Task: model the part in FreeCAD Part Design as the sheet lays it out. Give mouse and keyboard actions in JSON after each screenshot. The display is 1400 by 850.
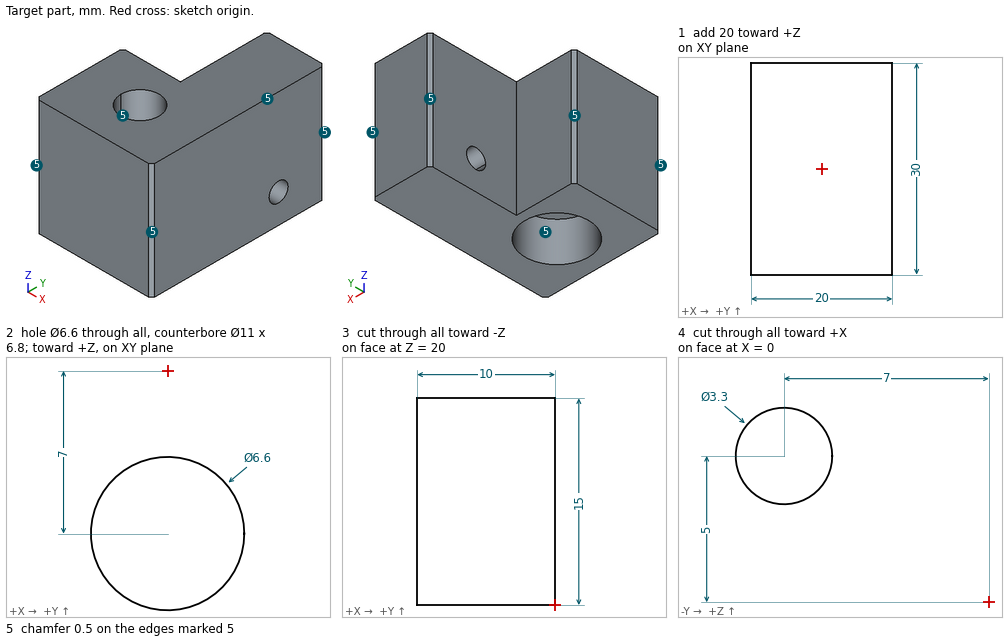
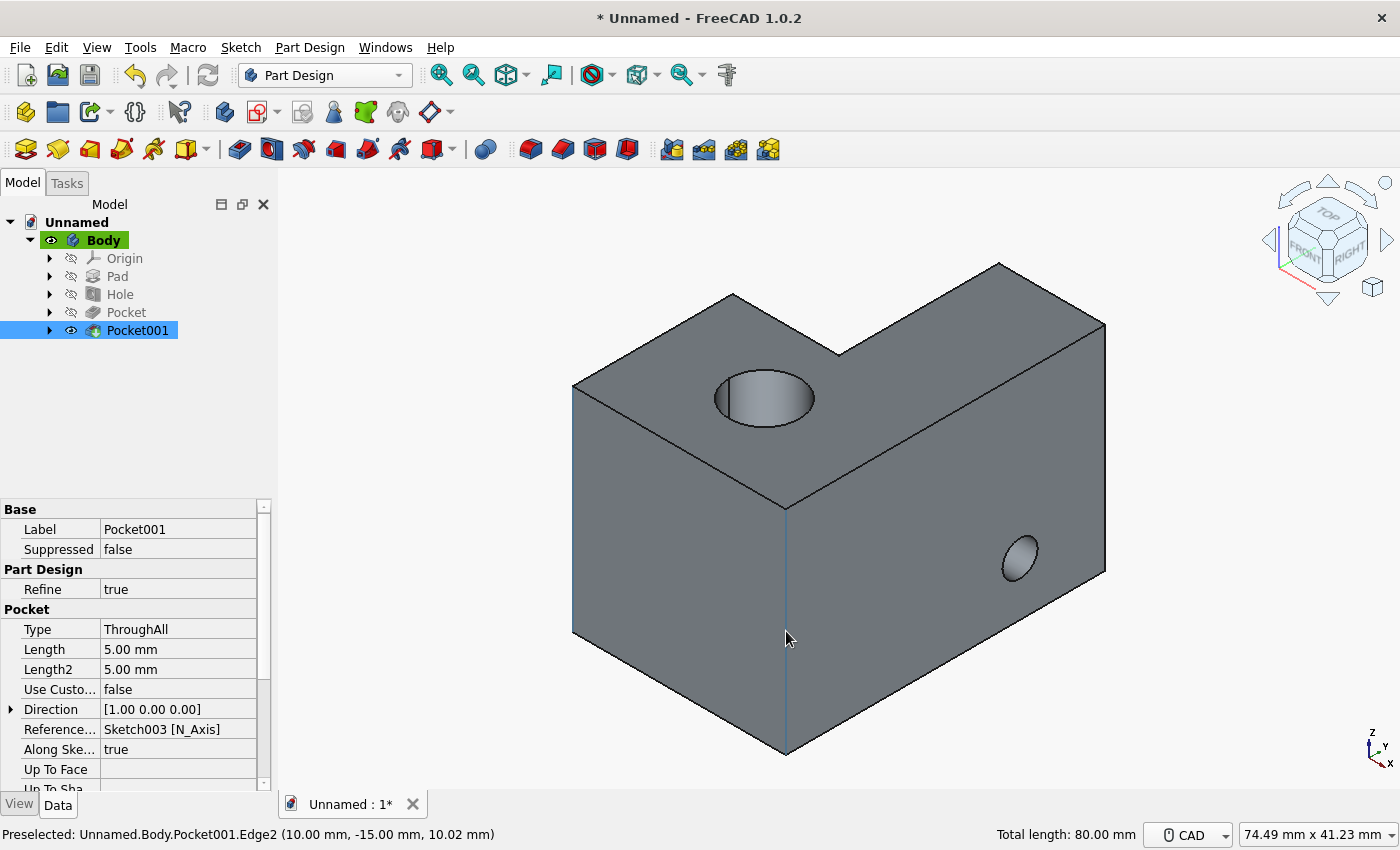
{"action": "key", "text": "2"}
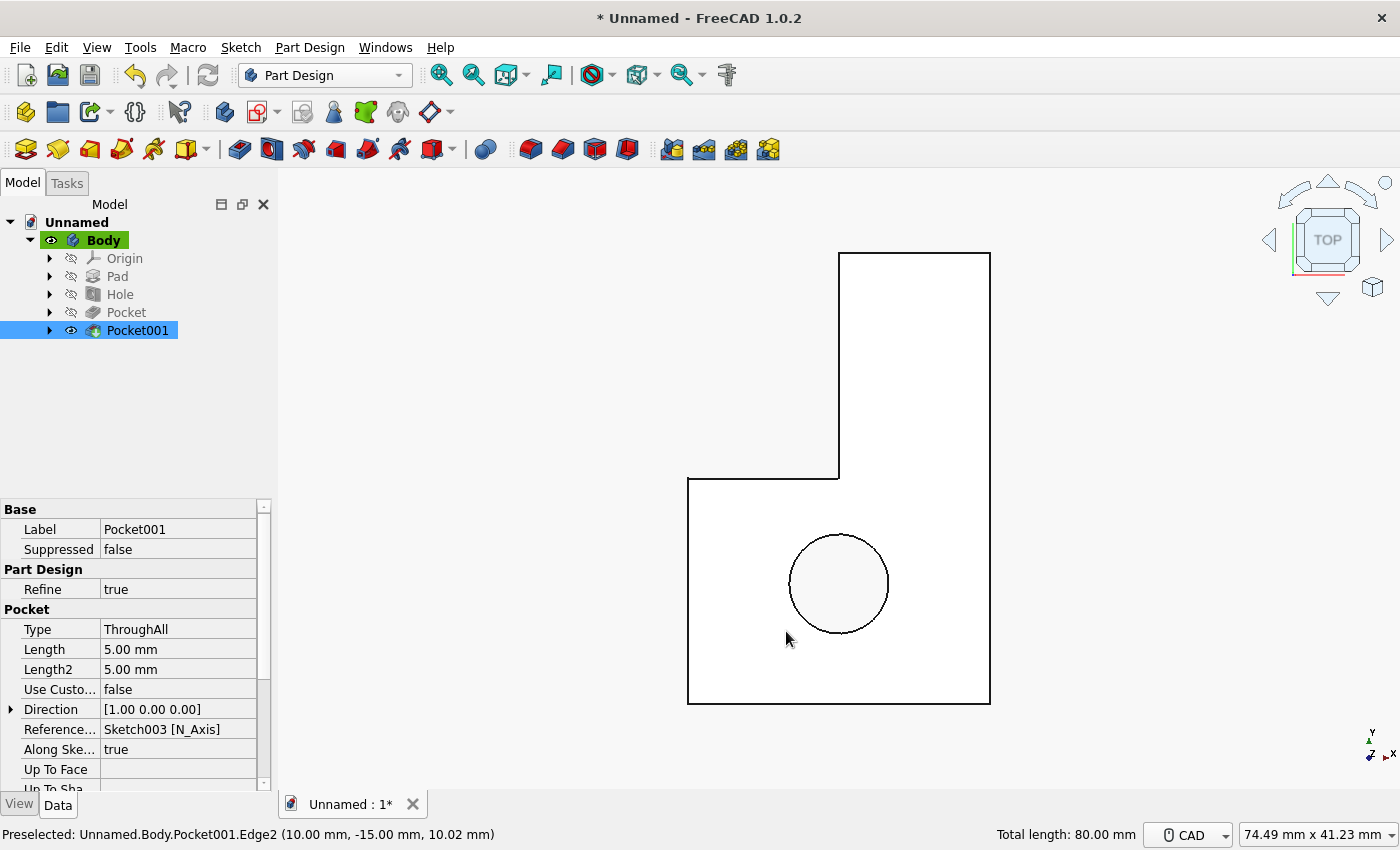
{"action": "key", "text": "1"}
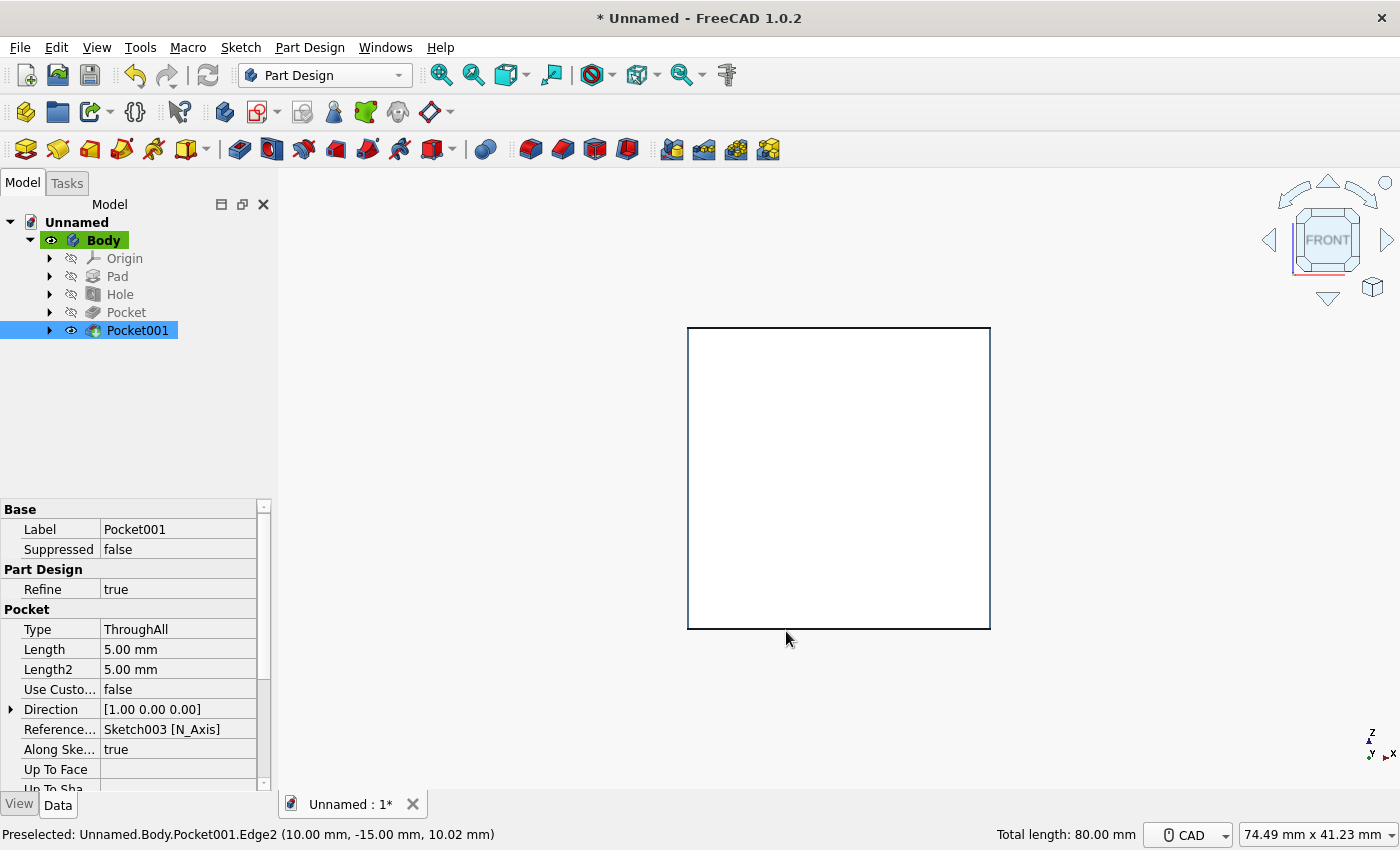
{"action": "key", "text": "3"}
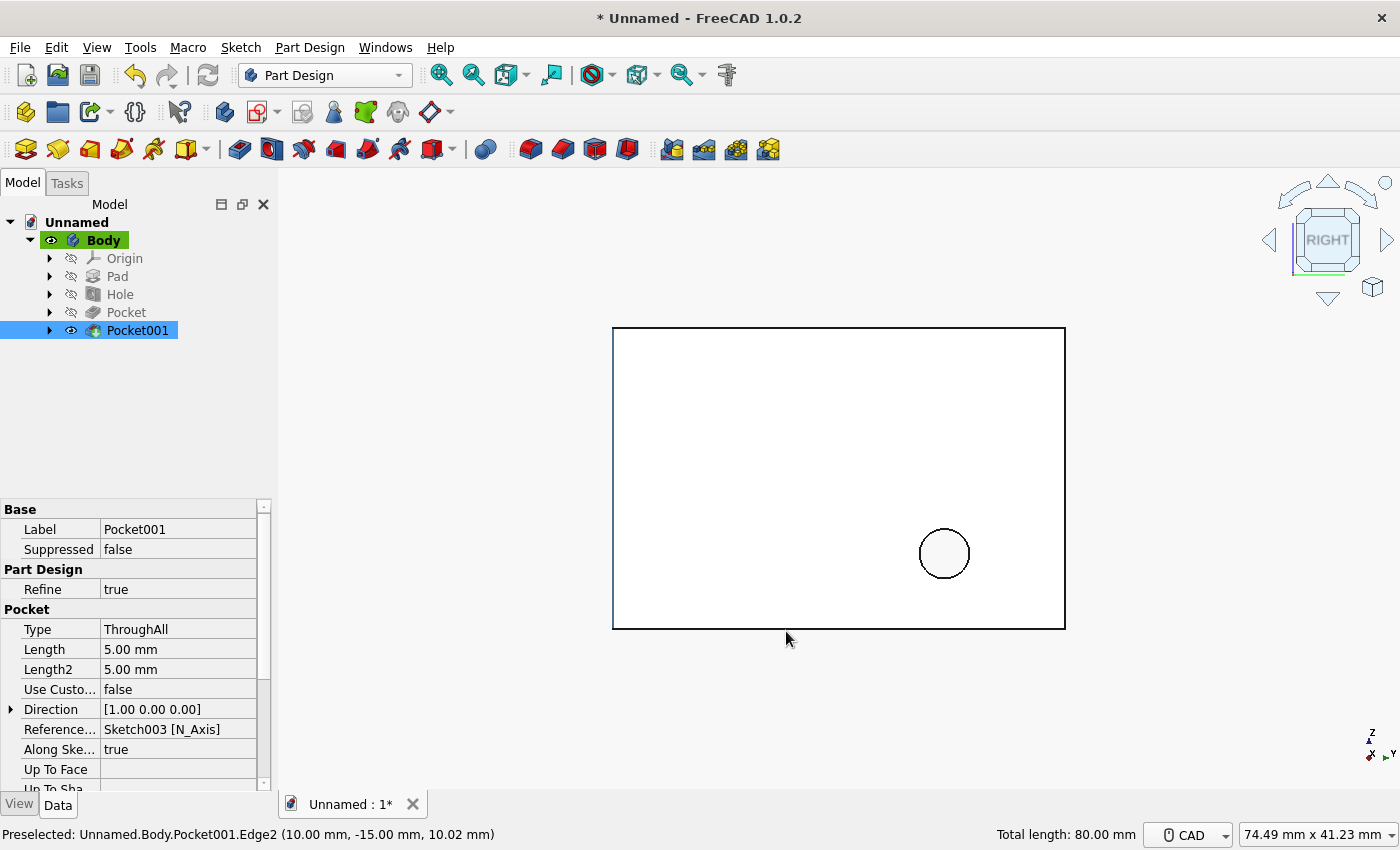
{"action": "left_click", "coordinate": [1065, 478], "text": "ctrl"}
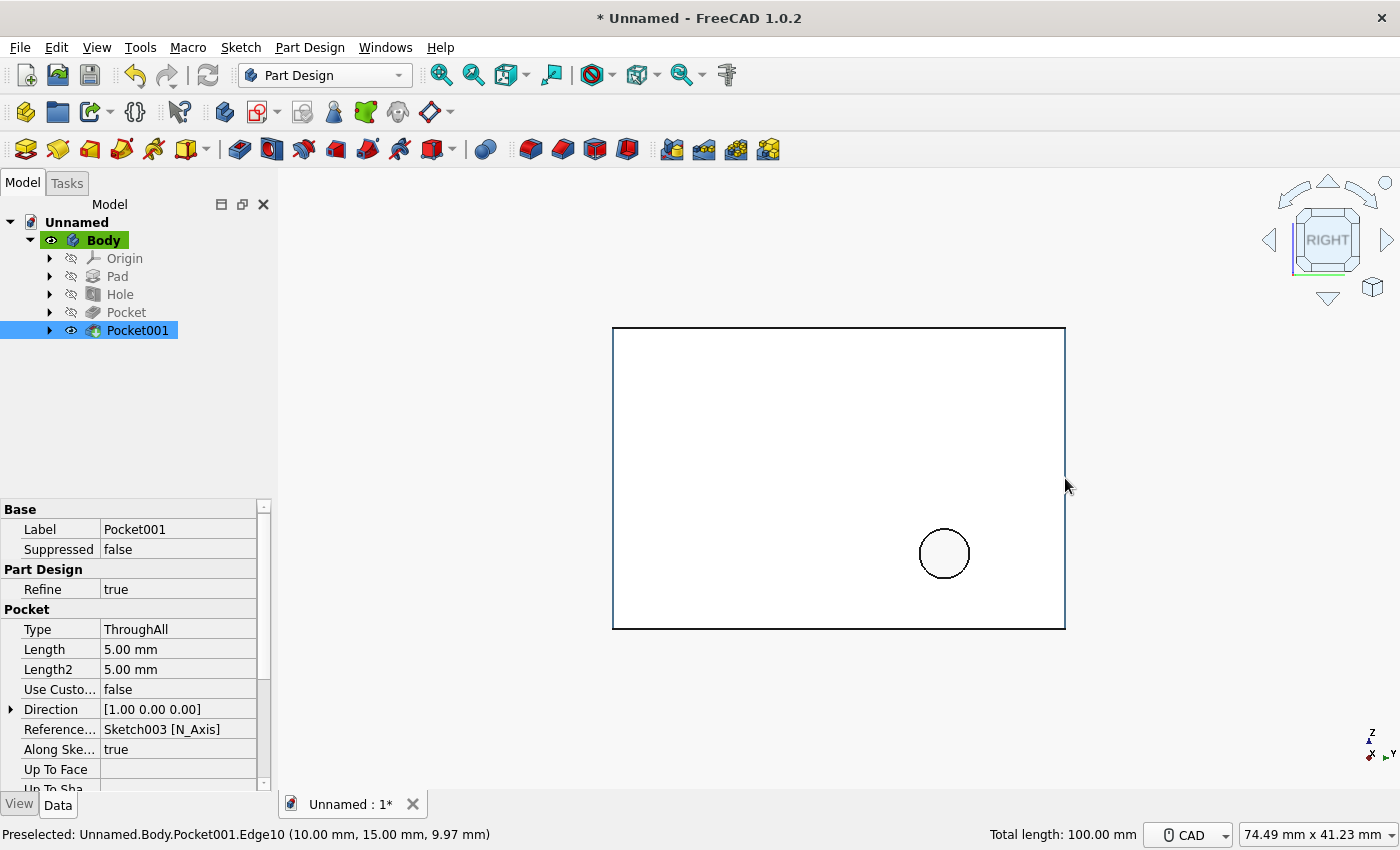
{"action": "left_click", "coordinate": [564, 150]}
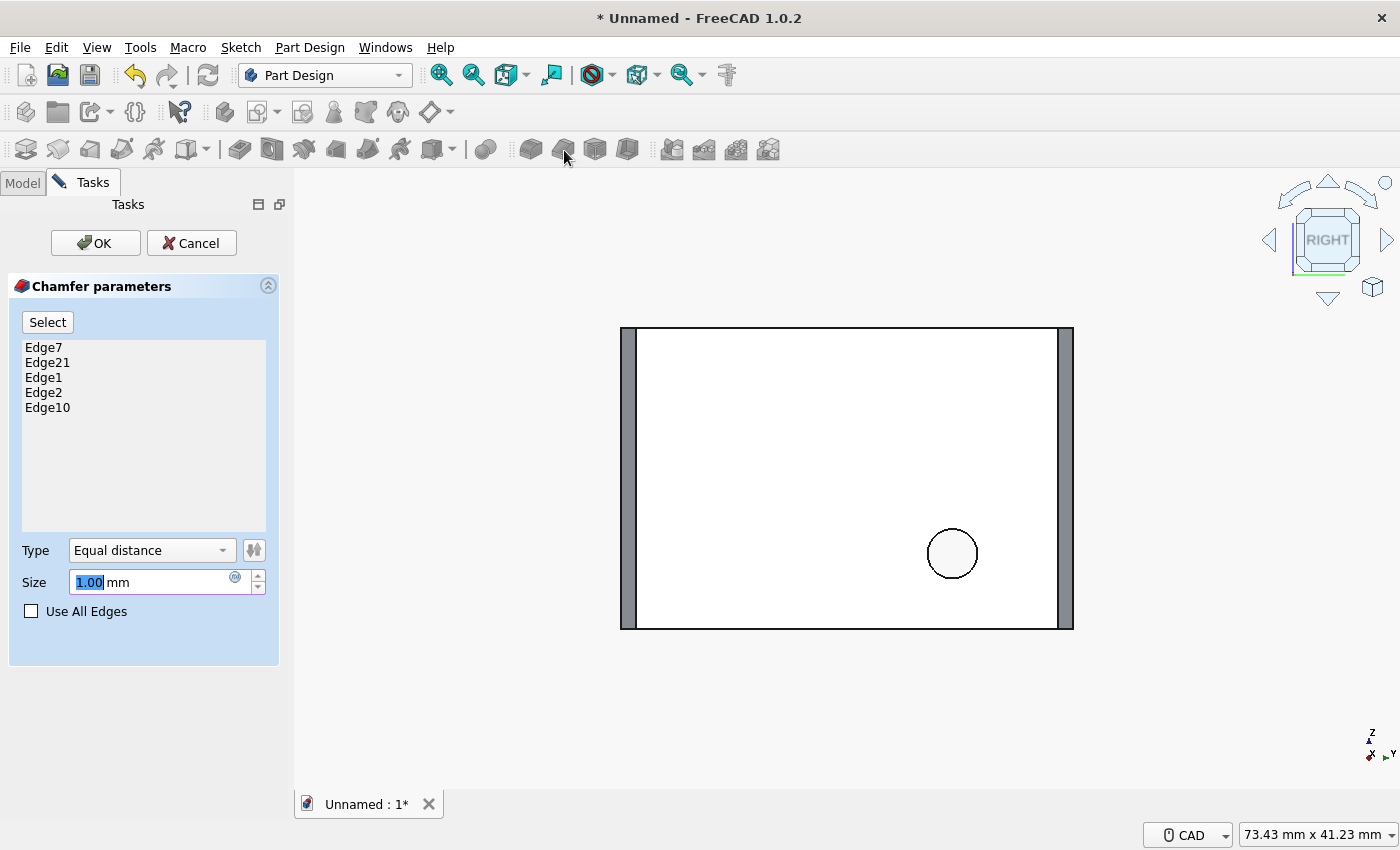
{"action": "type", "text": "0.5"}
{"action": "key", "text": "Tab"}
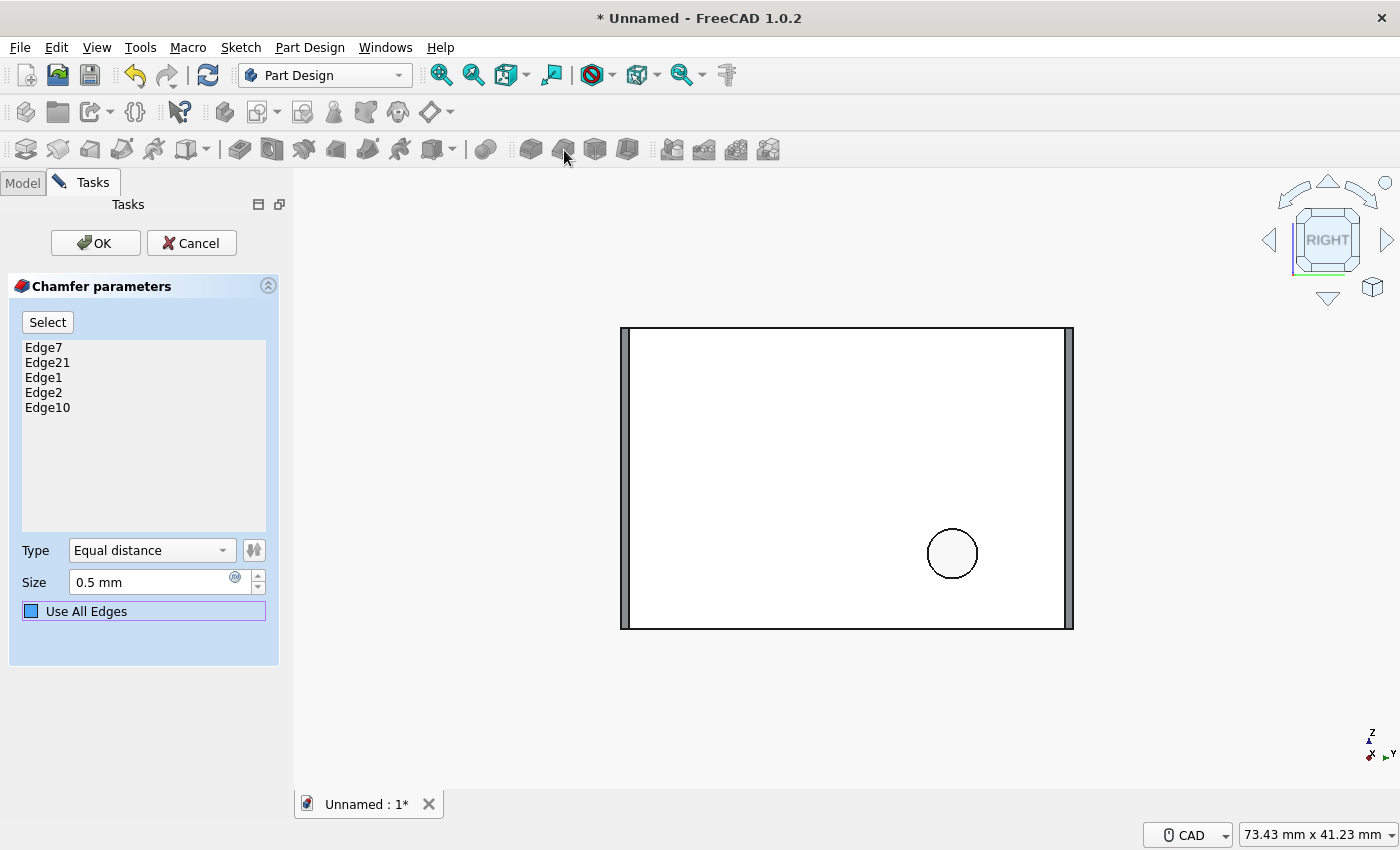
{"action": "left_click", "coordinate": [96, 243]}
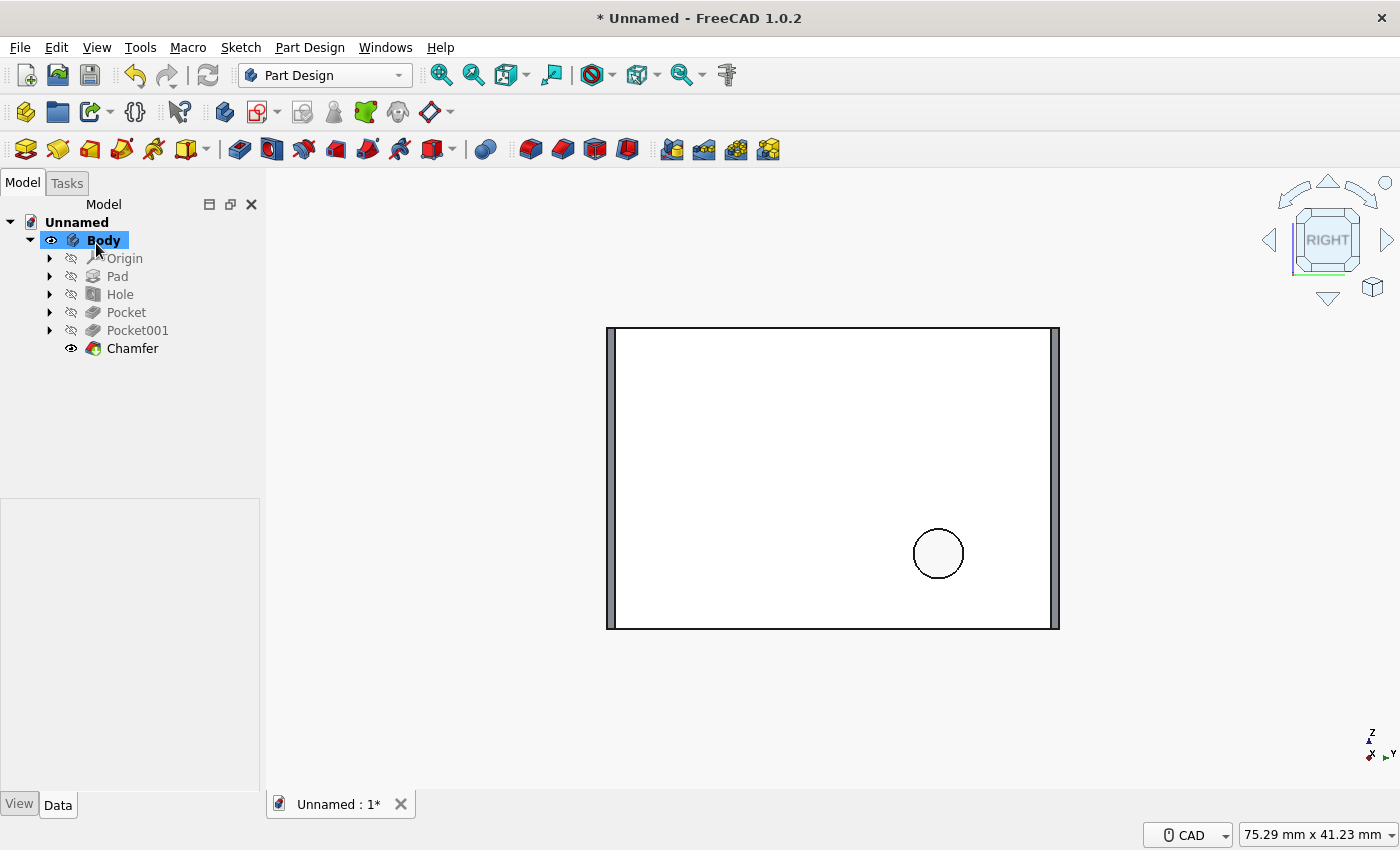
{"action": "key", "text": "0"}